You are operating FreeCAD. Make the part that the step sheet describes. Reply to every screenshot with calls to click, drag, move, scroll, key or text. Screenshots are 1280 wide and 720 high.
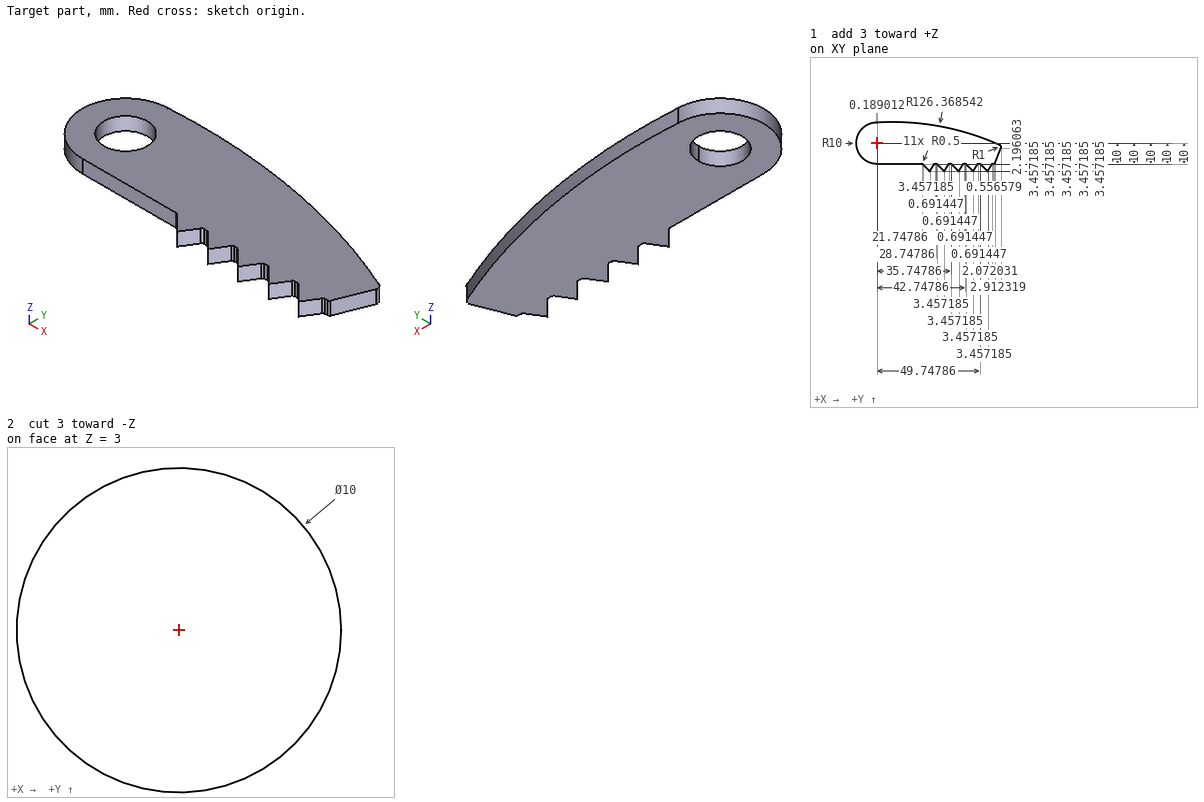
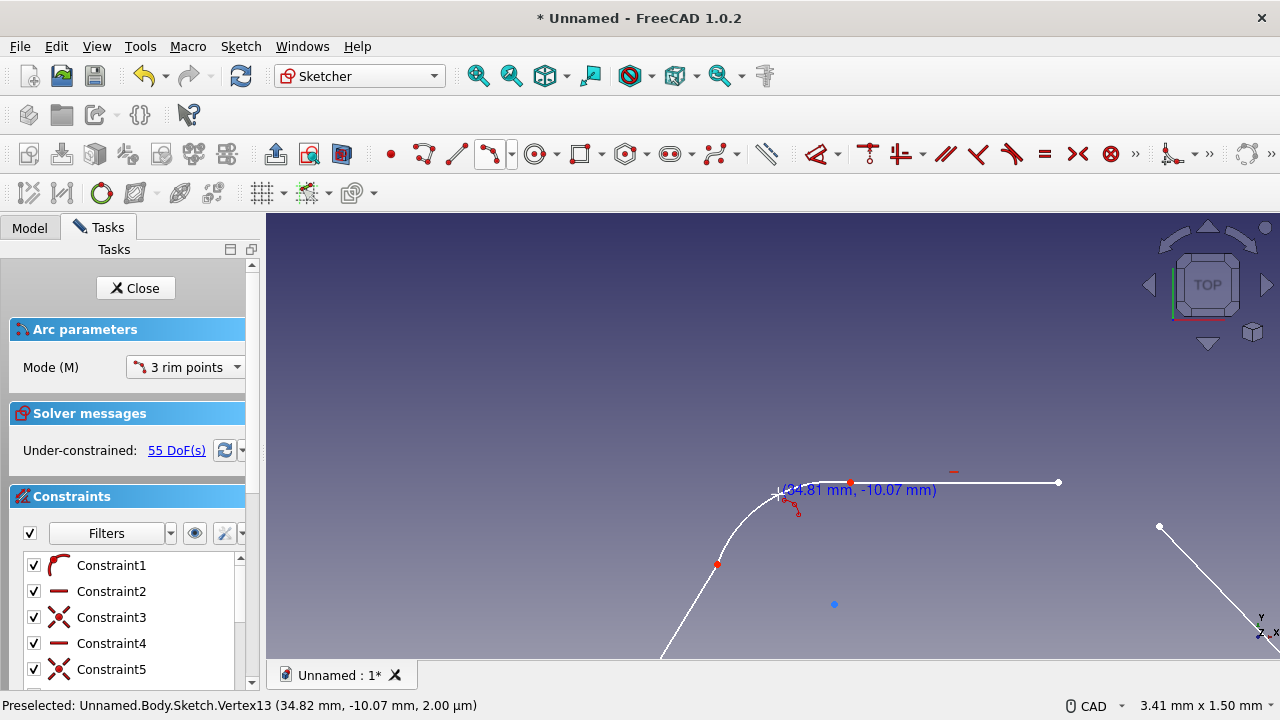
scroll(803, 519, down, 17)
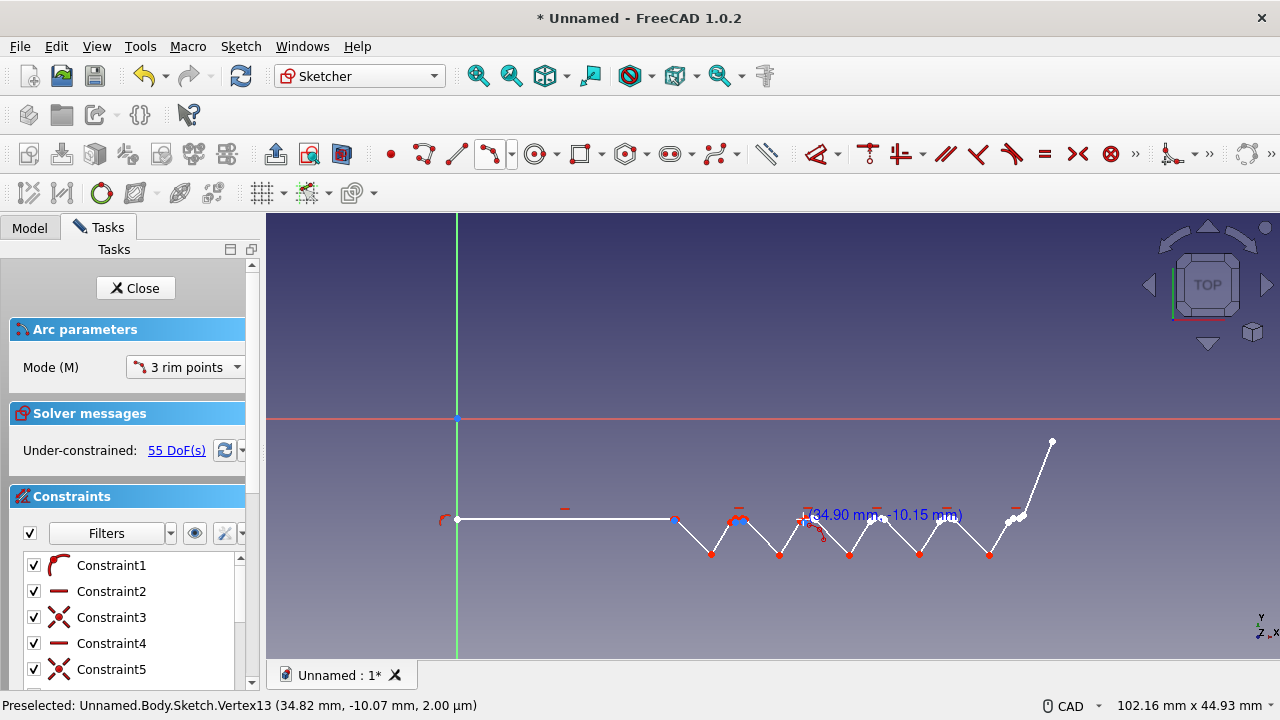
scroll(812, 518, up, 8)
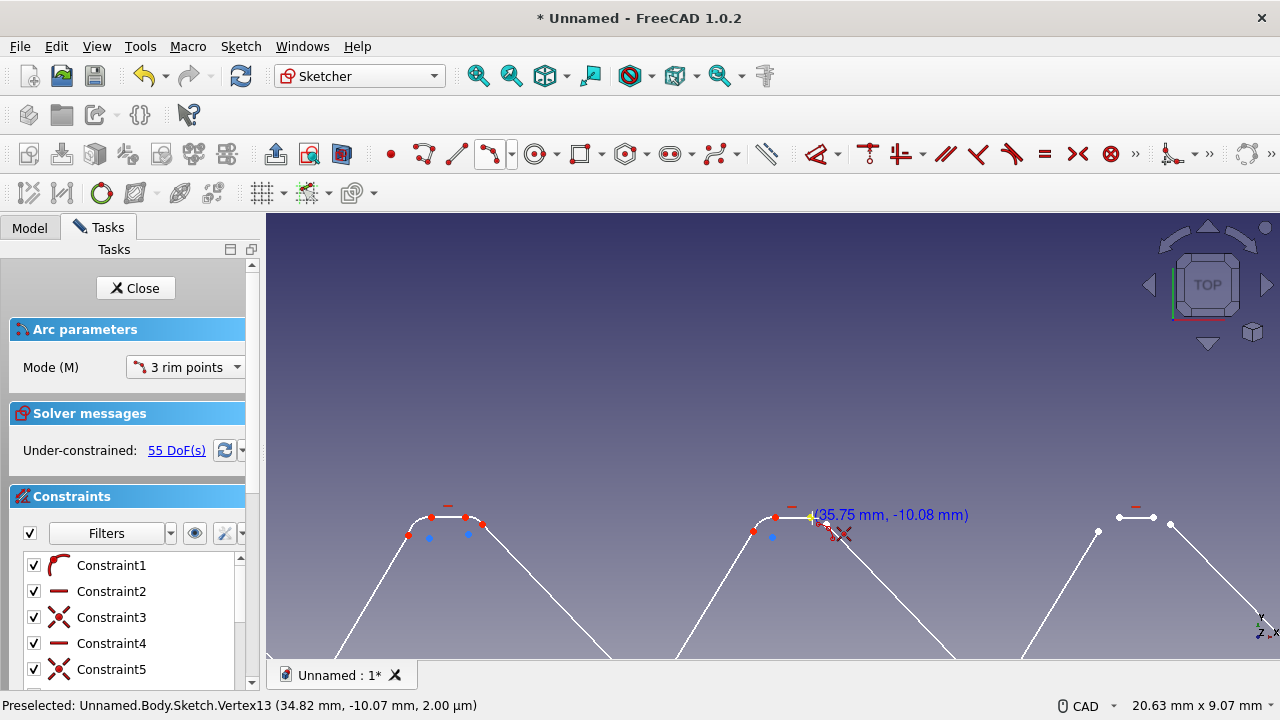
click(810, 518)
click(827, 525)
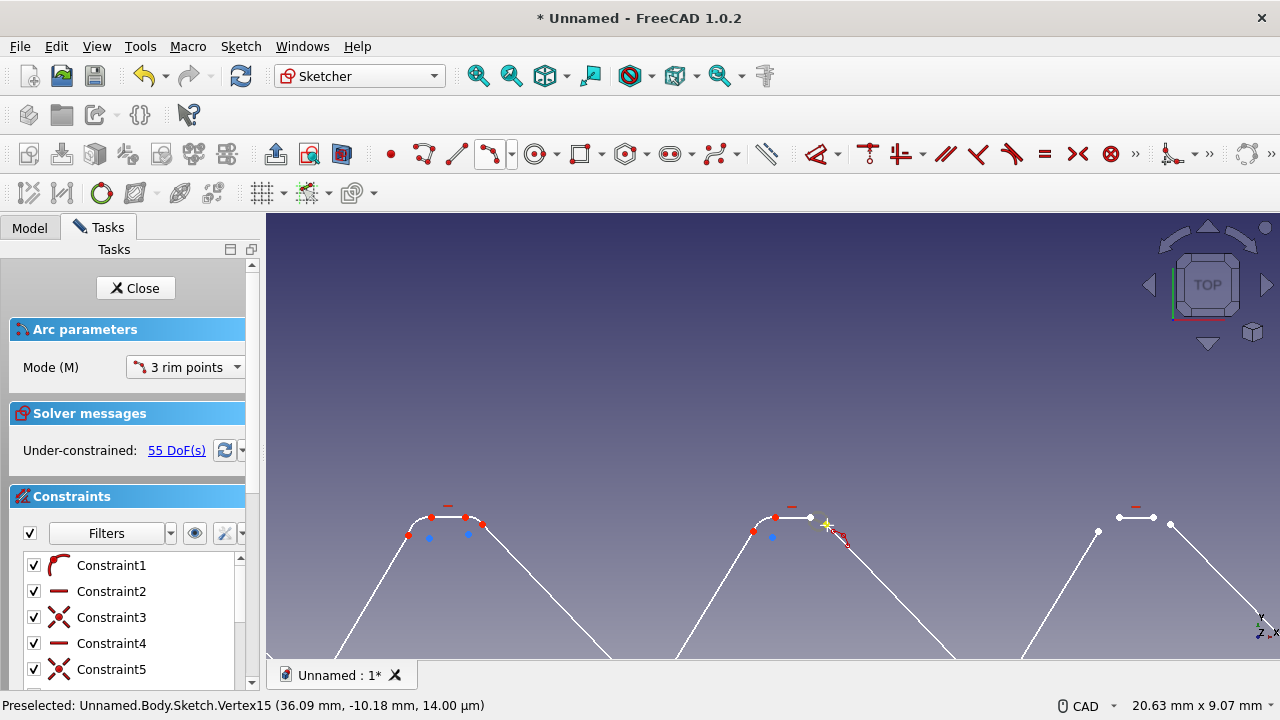
scroll(819, 518, up, 11)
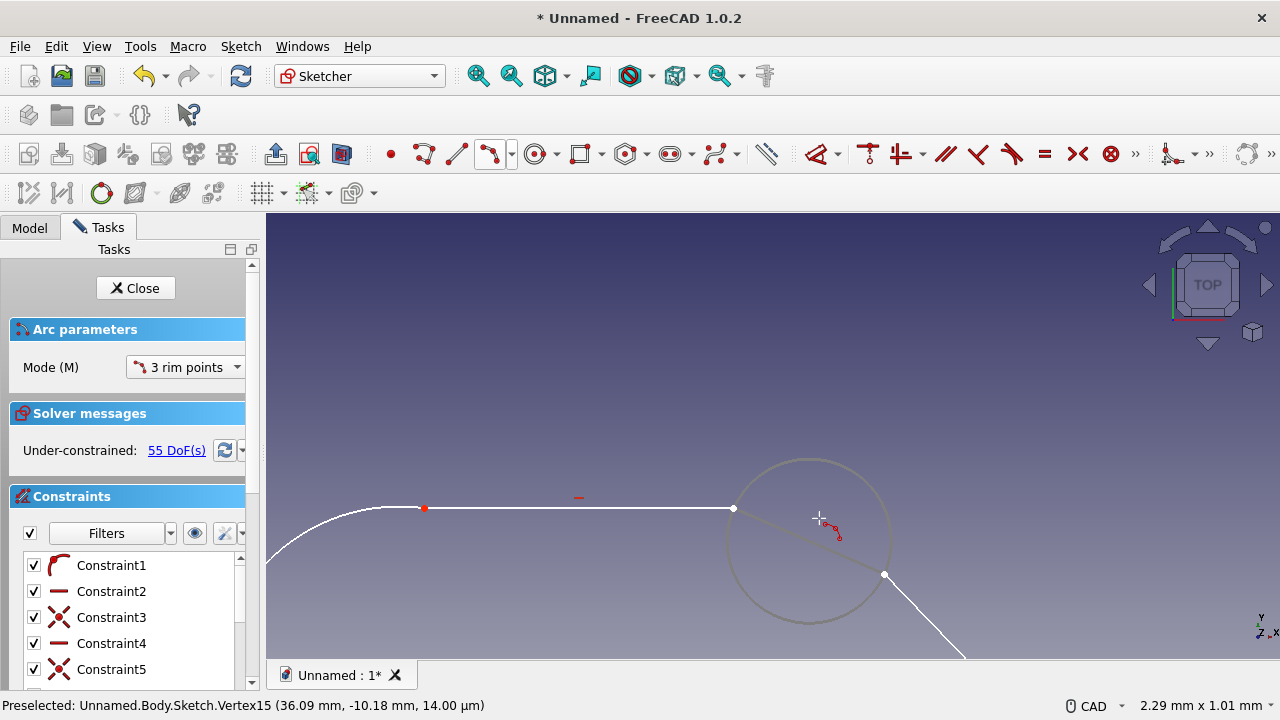
click(816, 513)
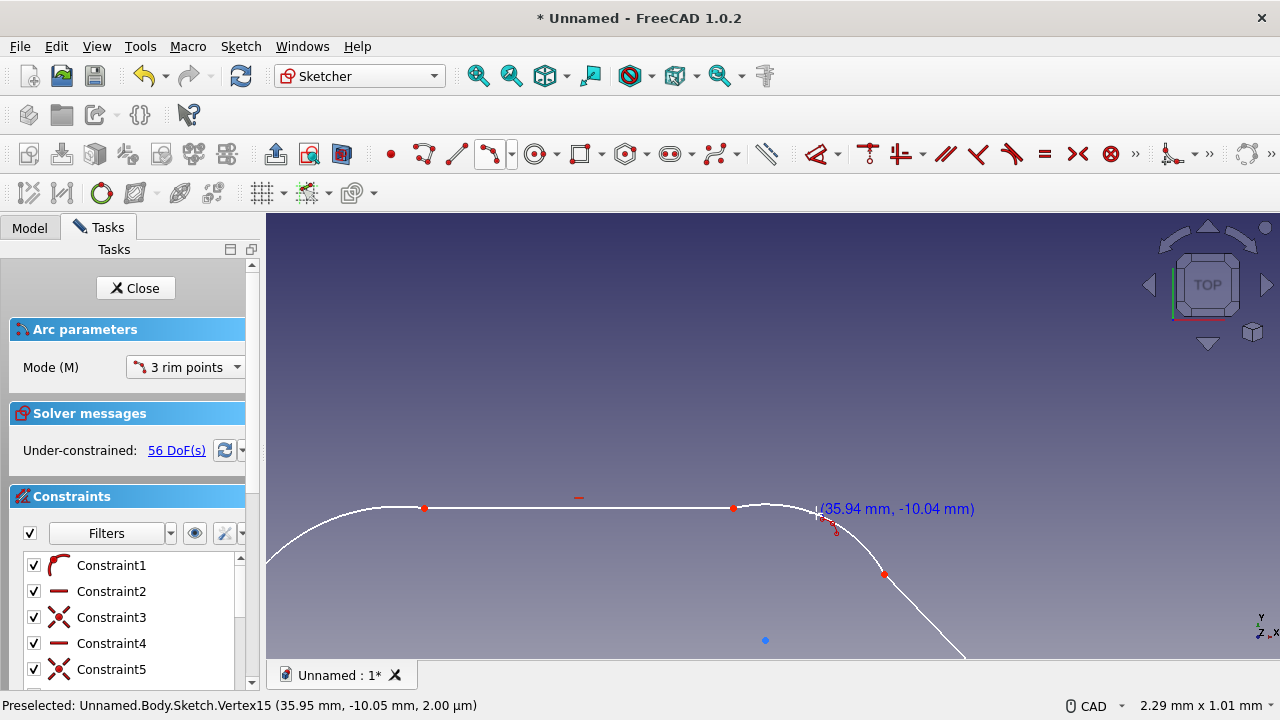
scroll(704, 436, down, 15)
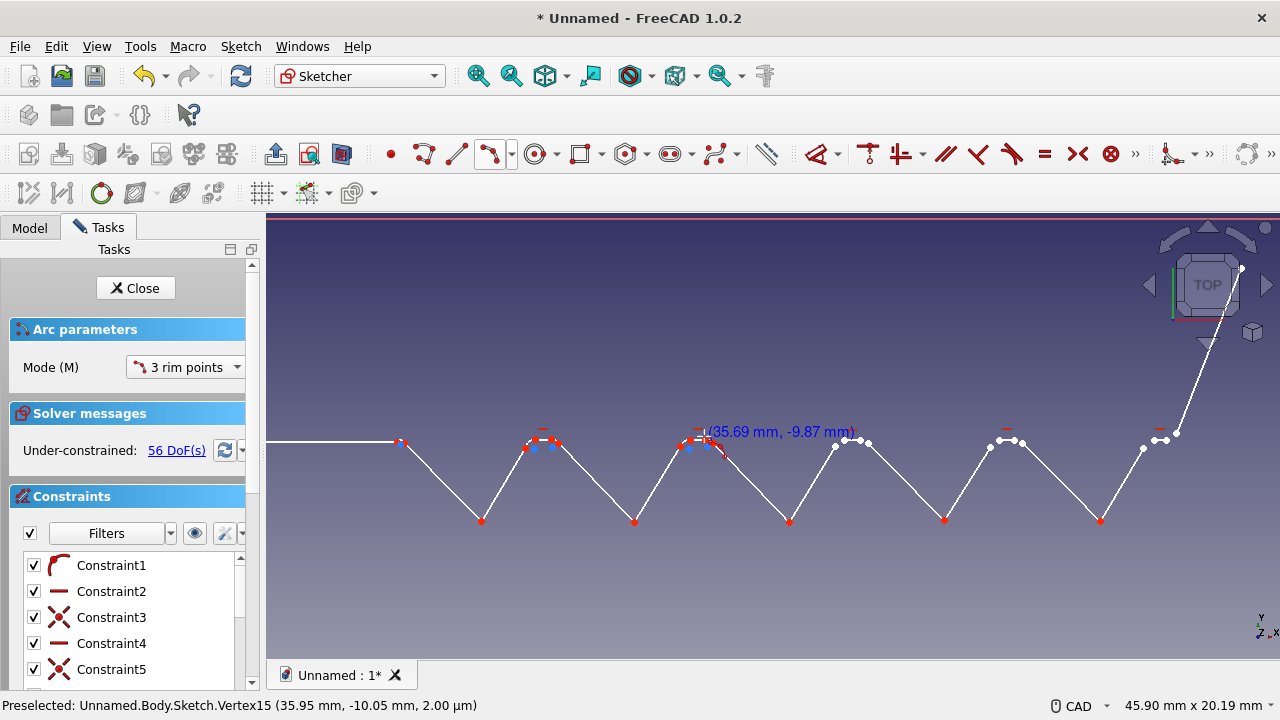
scroll(842, 539, down, 5)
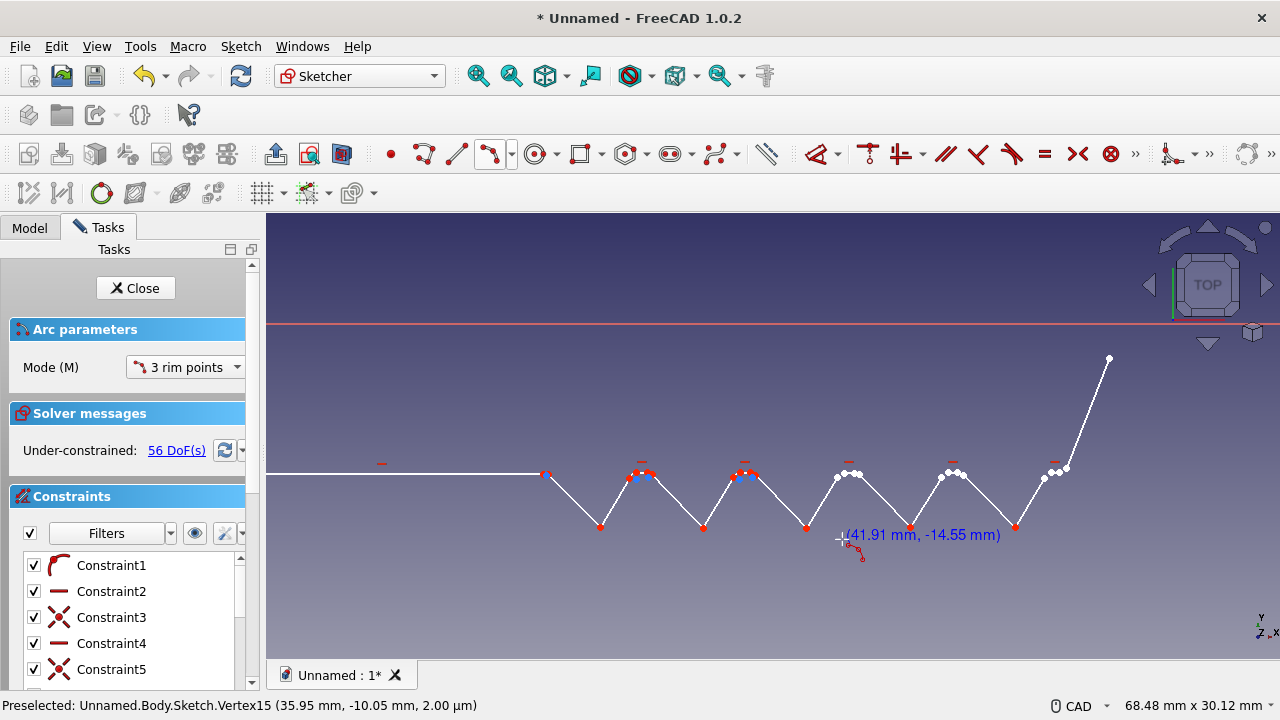
scroll(840, 505, up, 7)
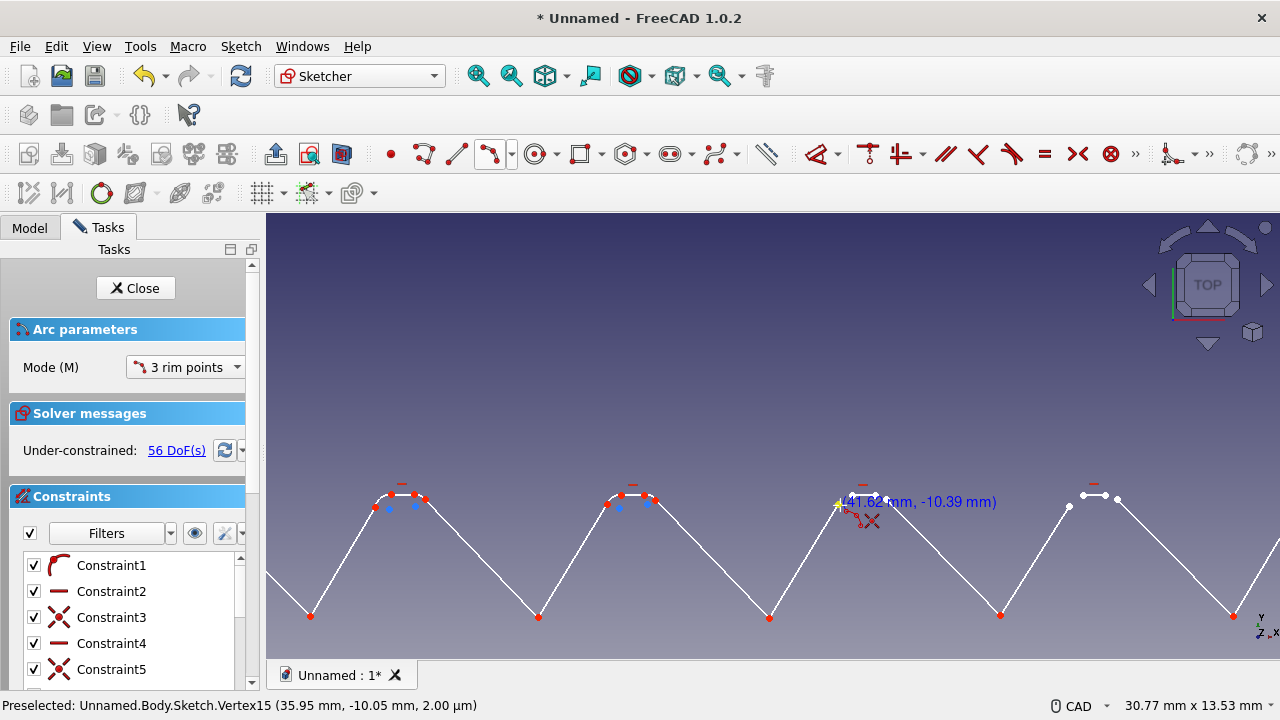
click(838, 505)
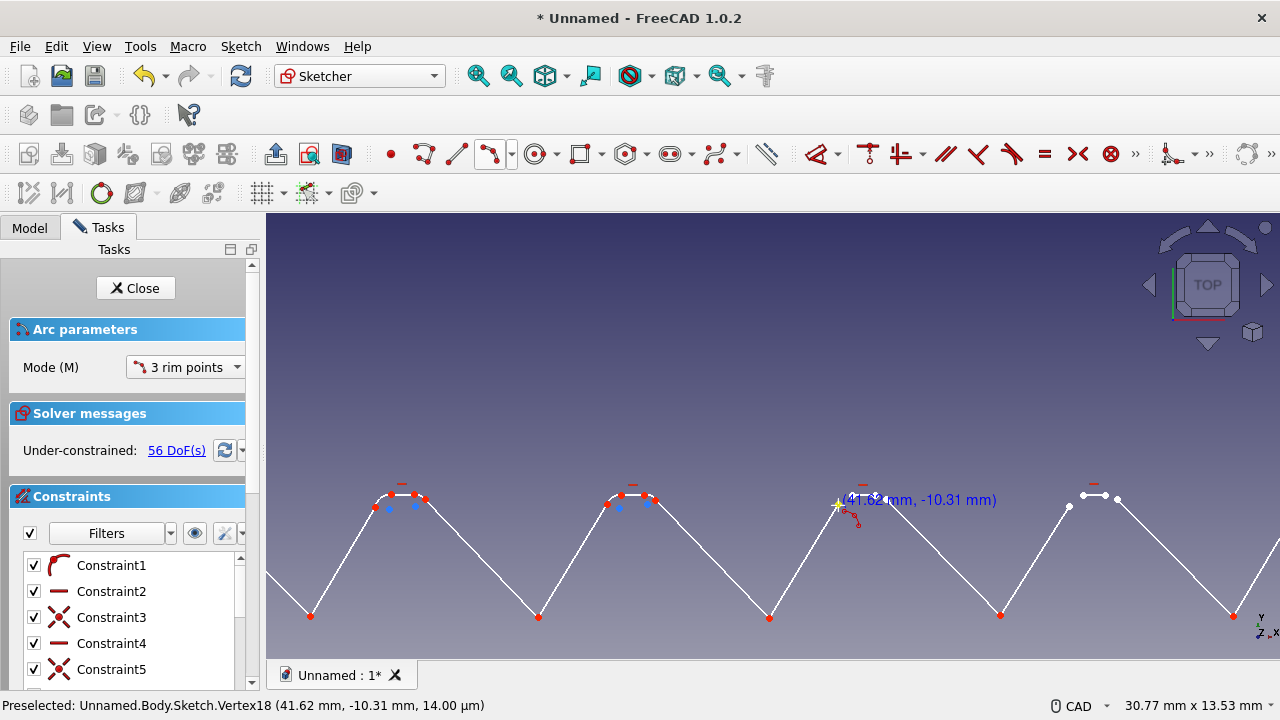
scroll(852, 494, up, 2)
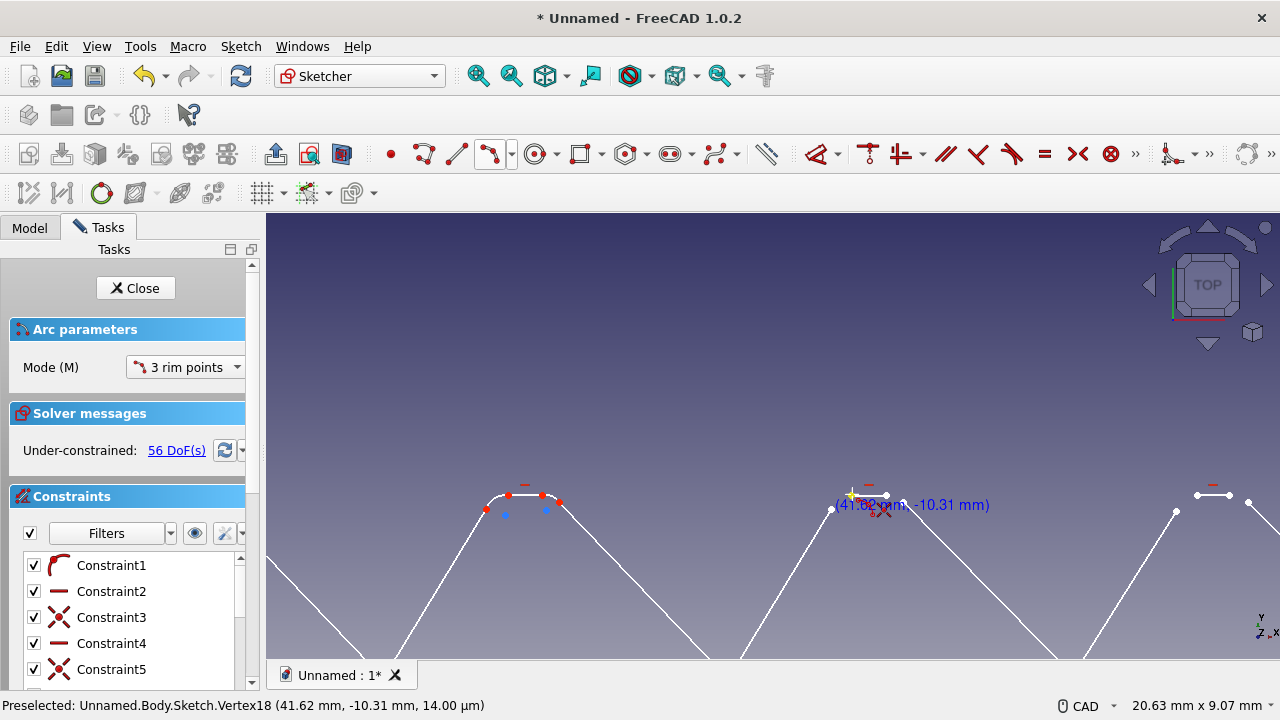
click(852, 496)